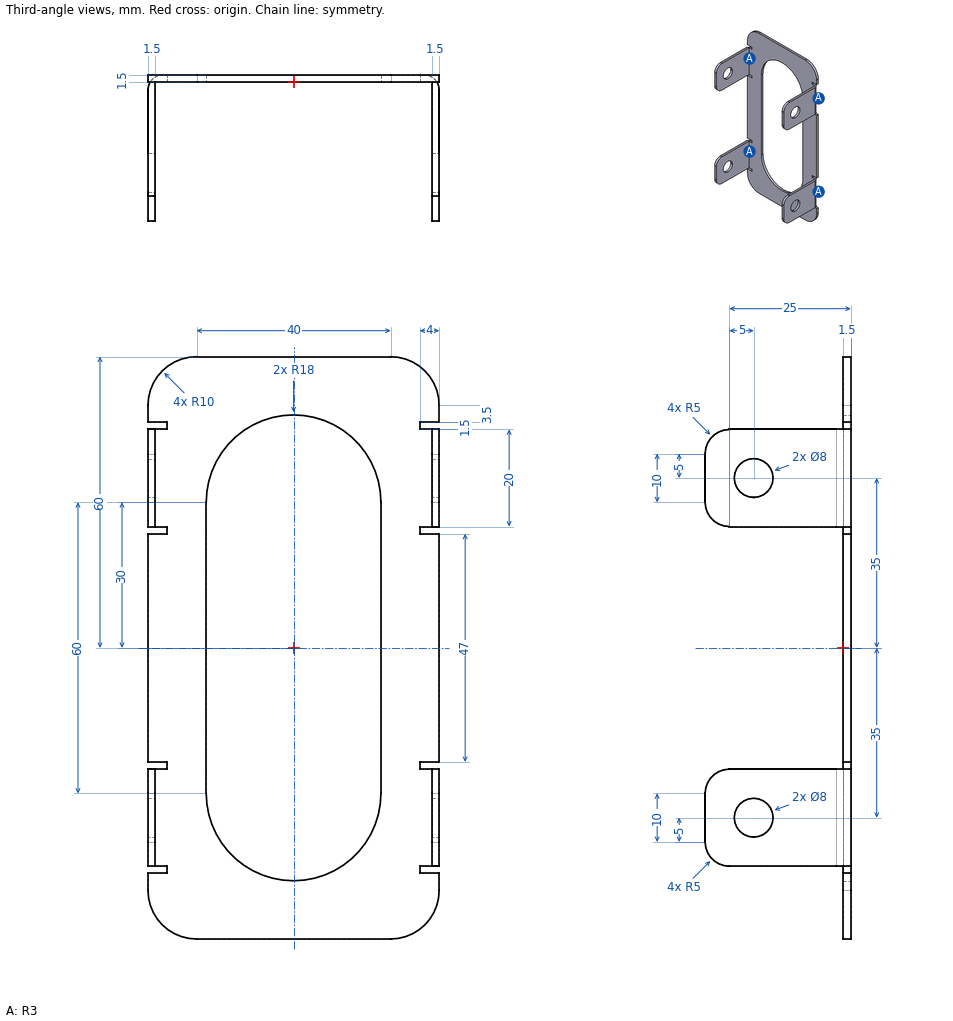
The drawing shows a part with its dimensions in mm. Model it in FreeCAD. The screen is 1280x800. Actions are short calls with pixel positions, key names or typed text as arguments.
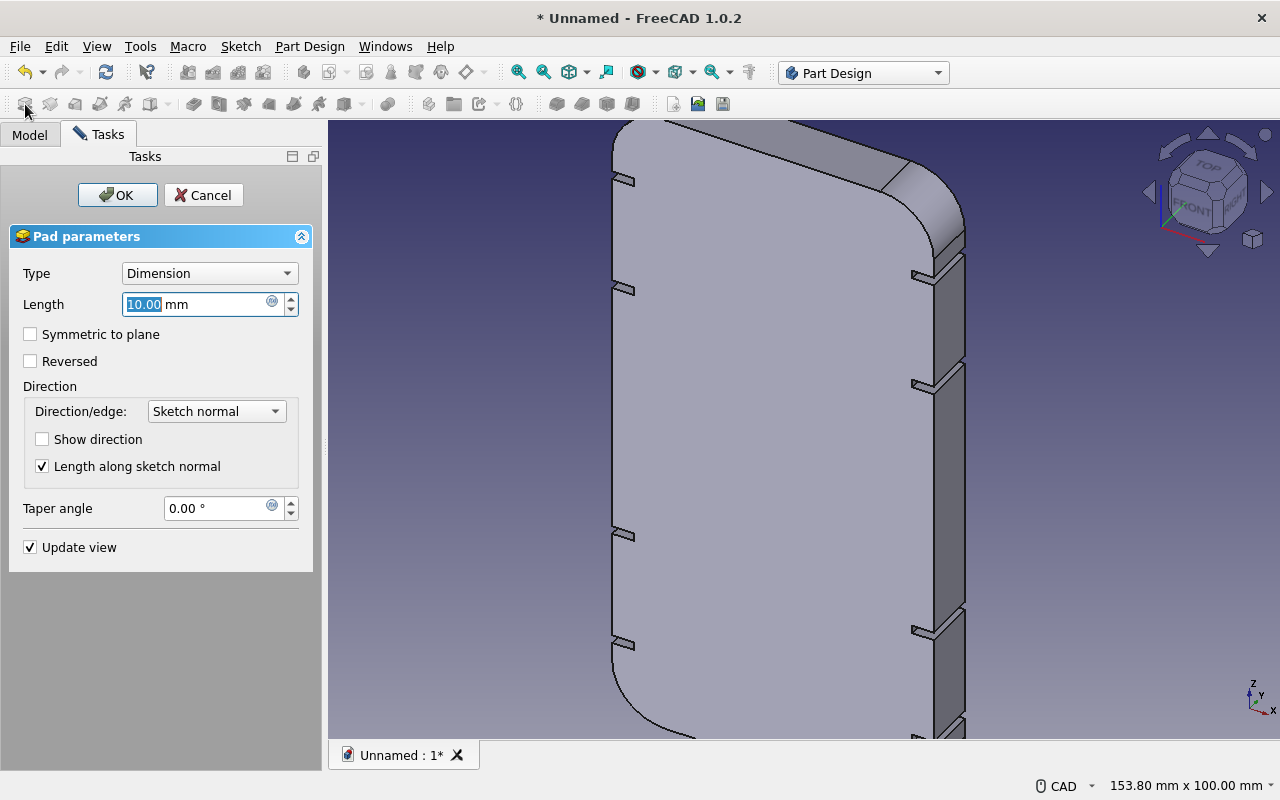
text(1.5)
key(Tab)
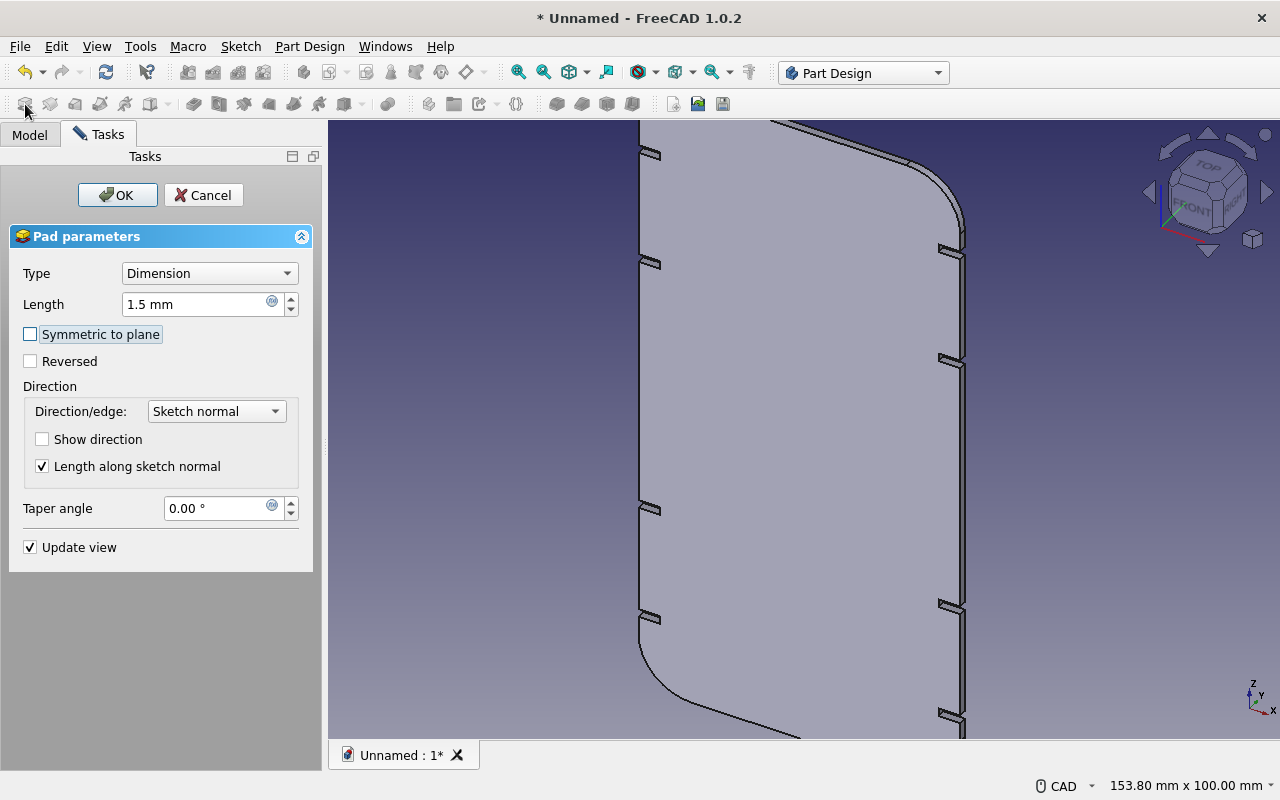
click(31, 361)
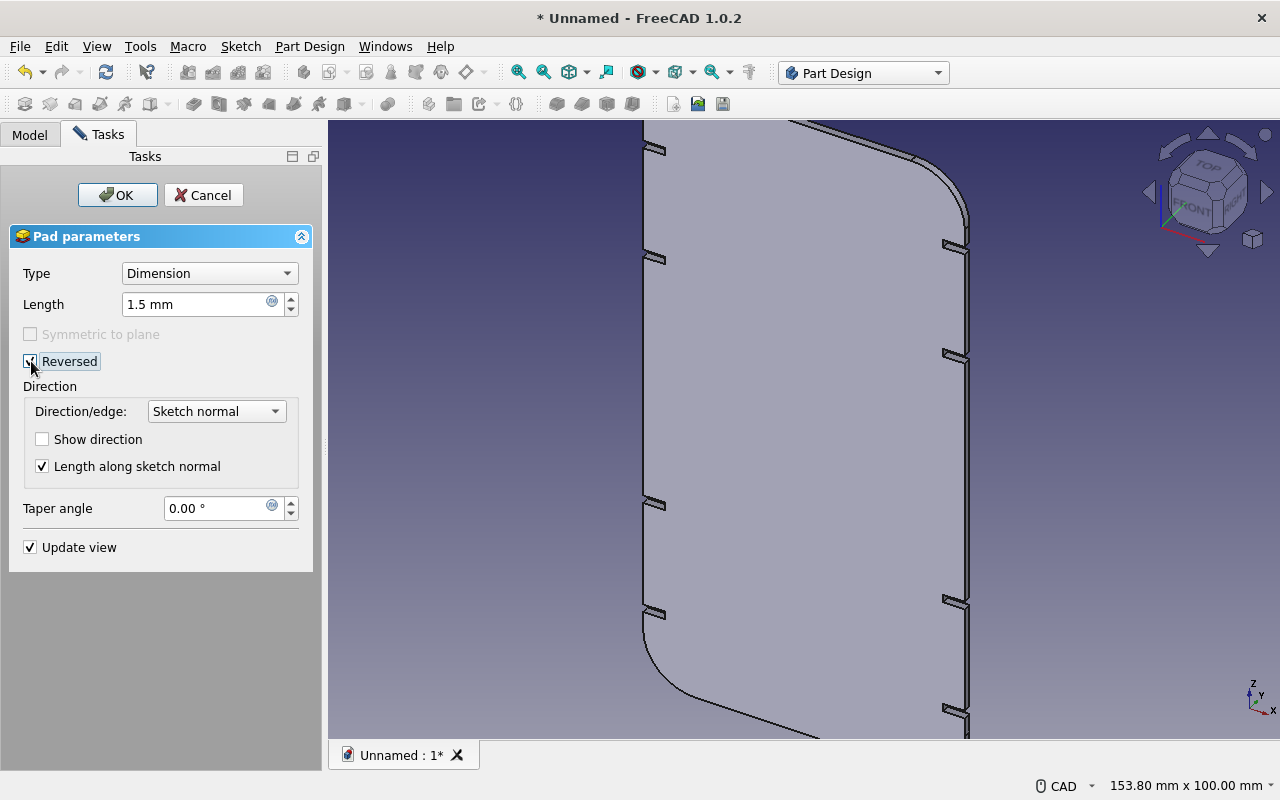
click(118, 195)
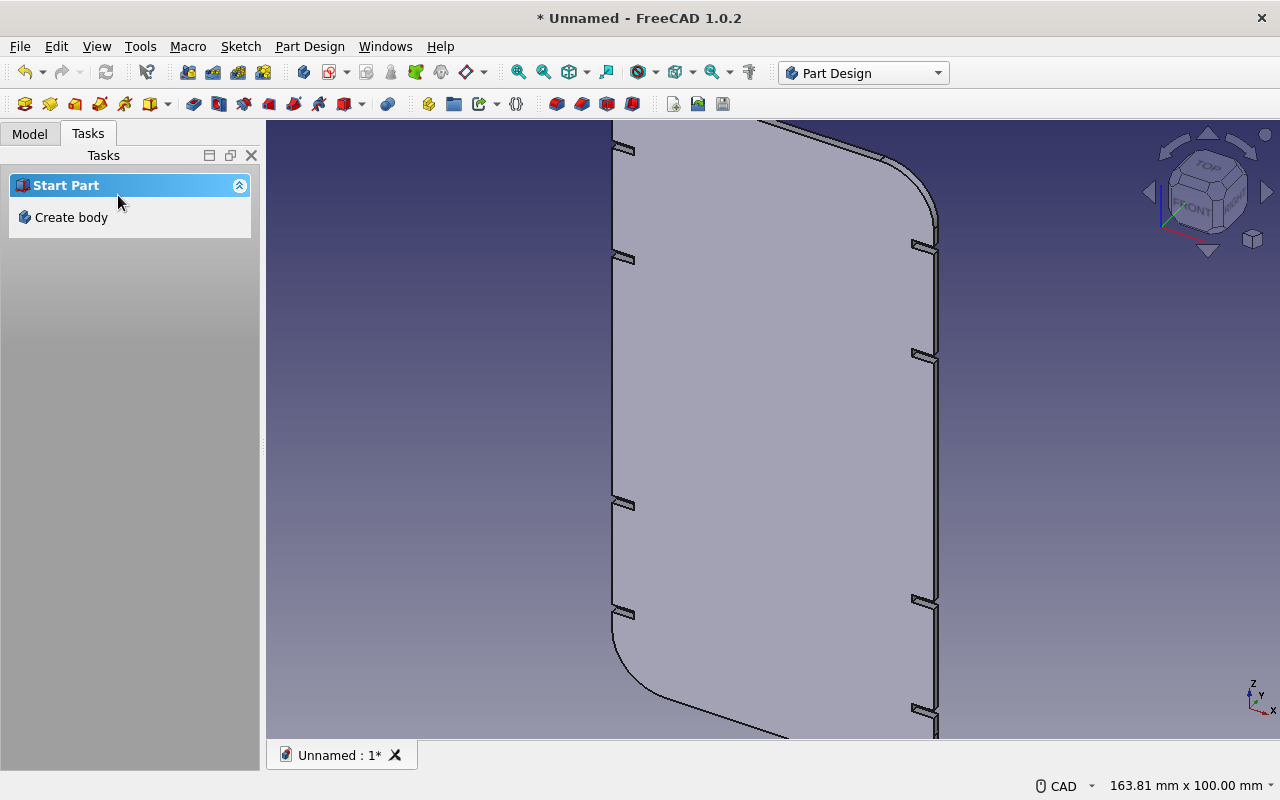
click(519, 72)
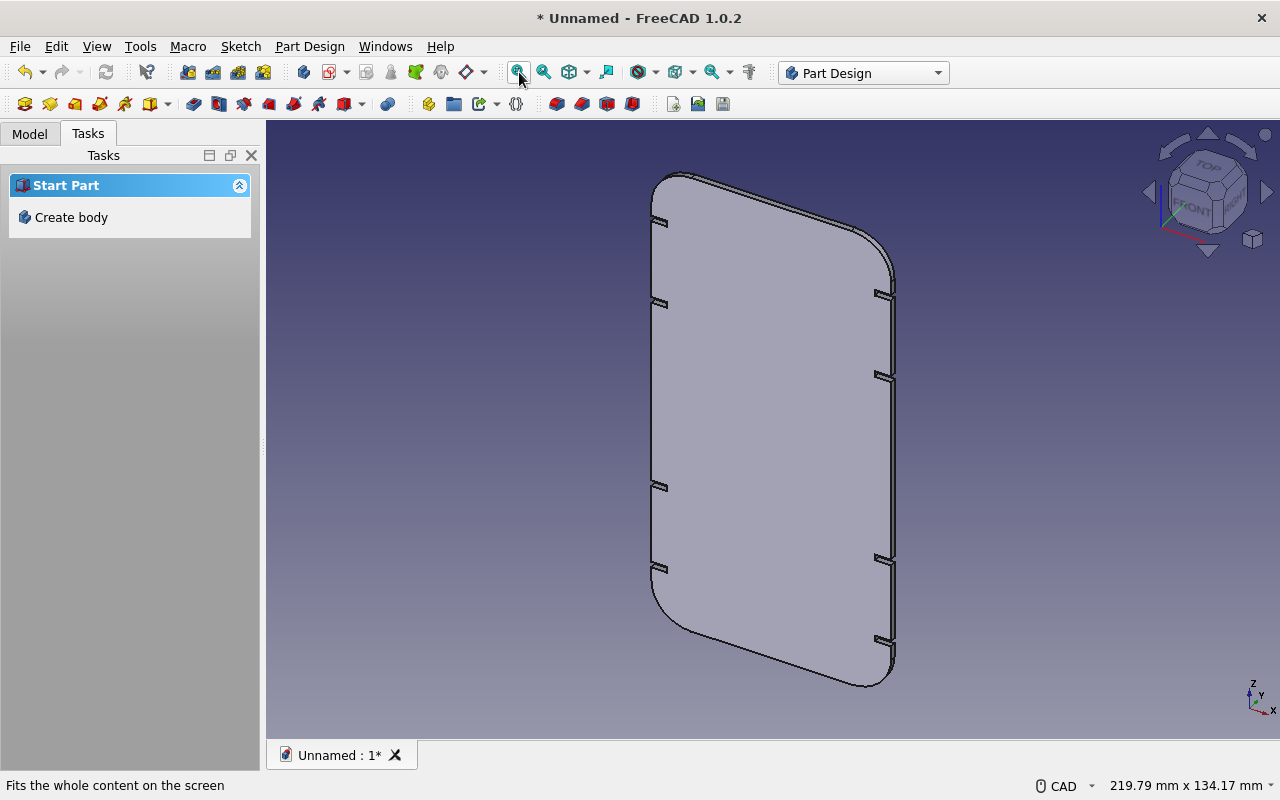
scroll(893, 392, up, 7)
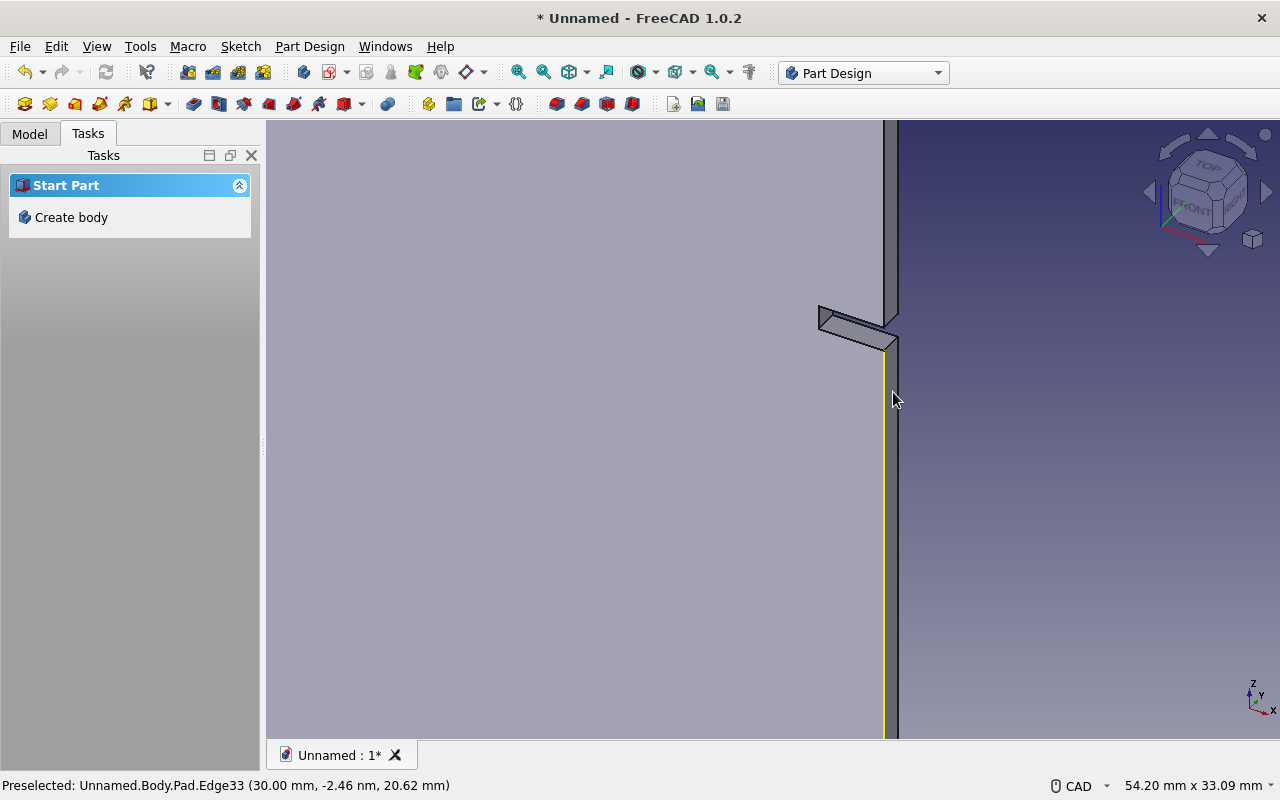
click(519, 72)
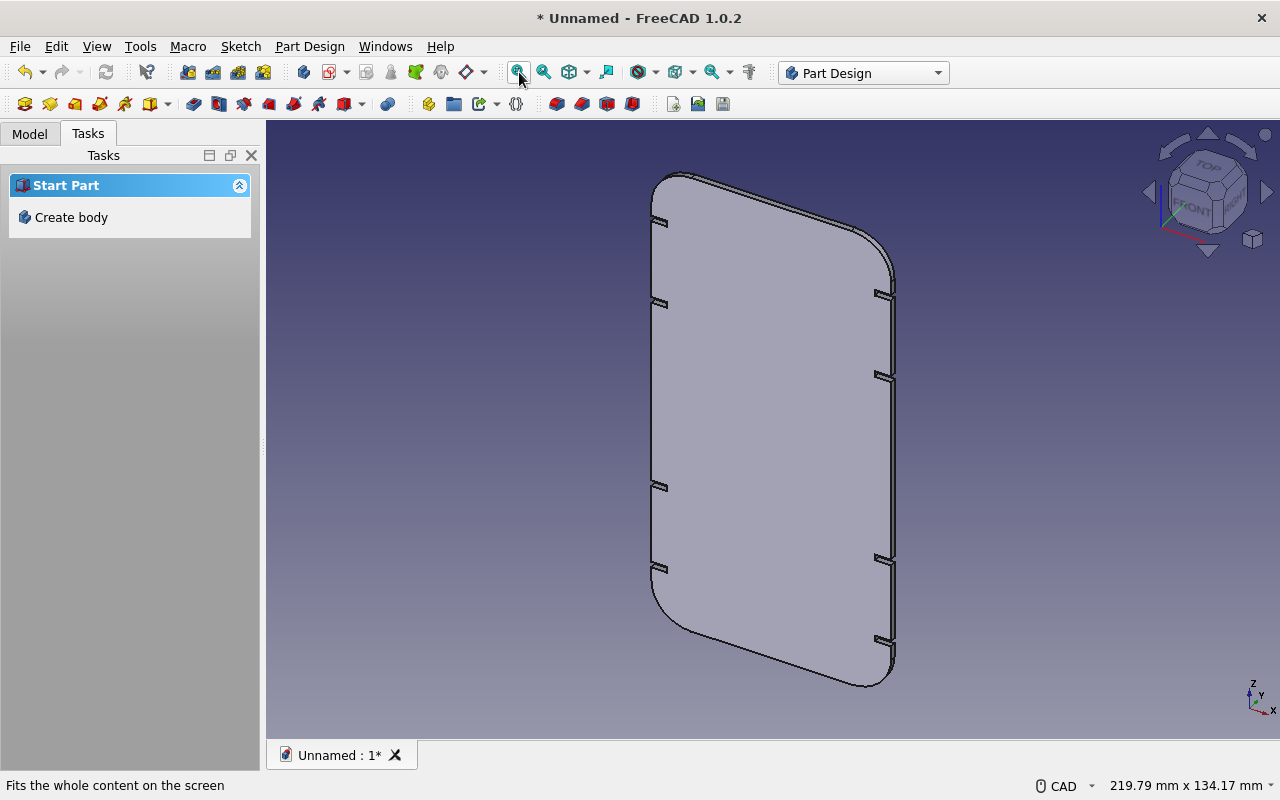
key(0)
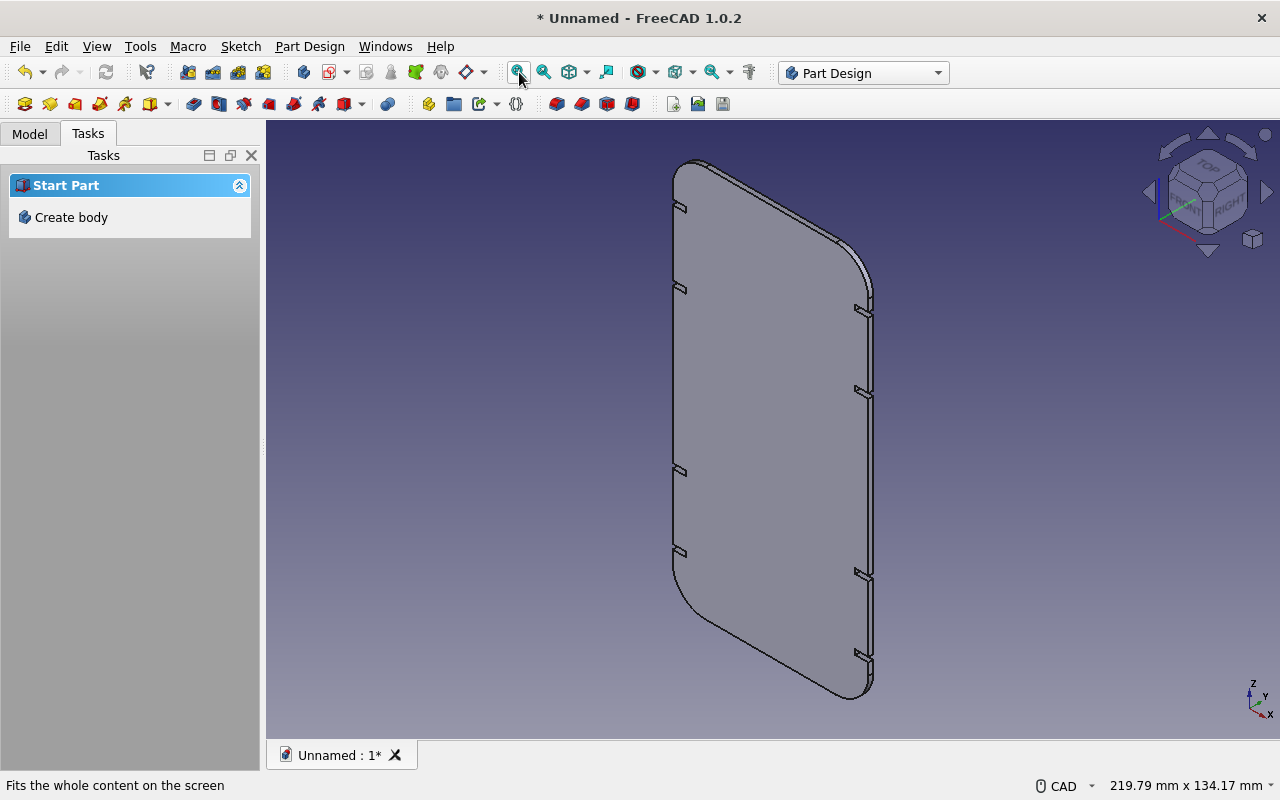
scroll(871, 409, up, 7)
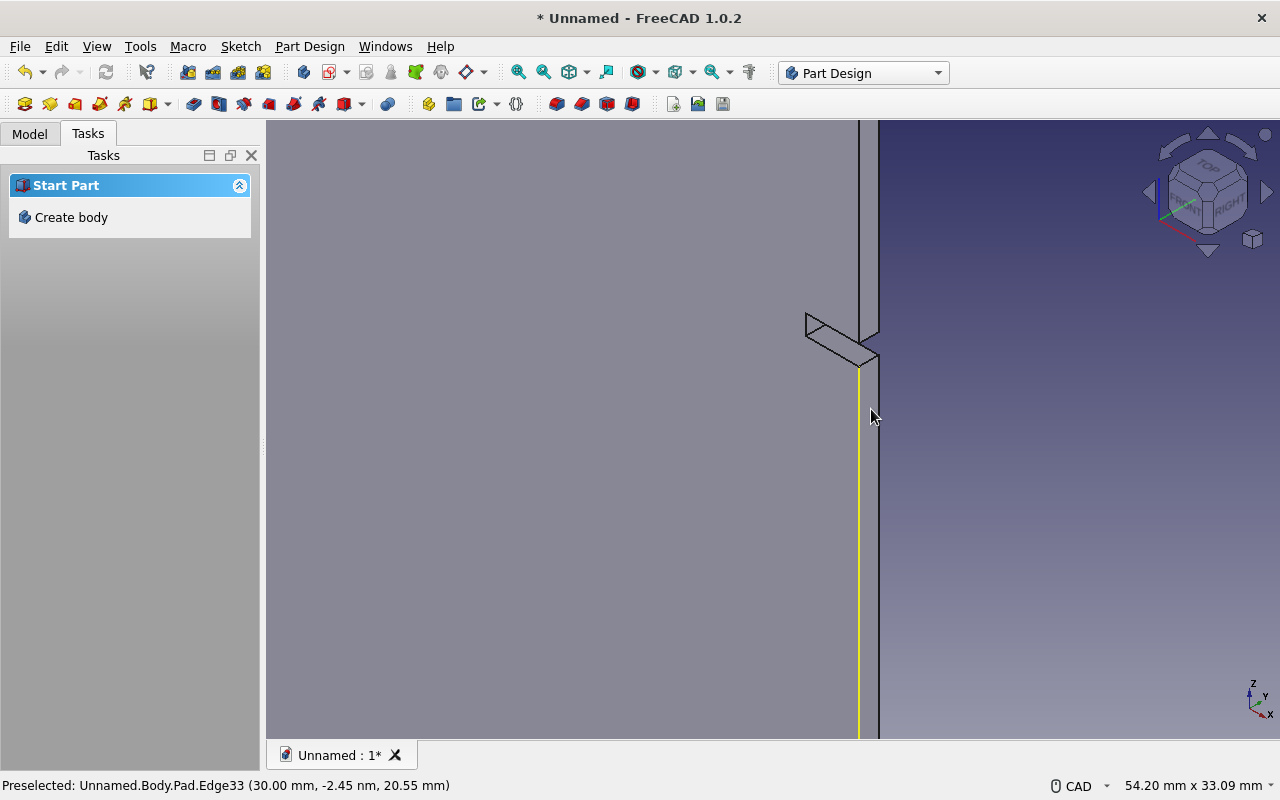
click(869, 411)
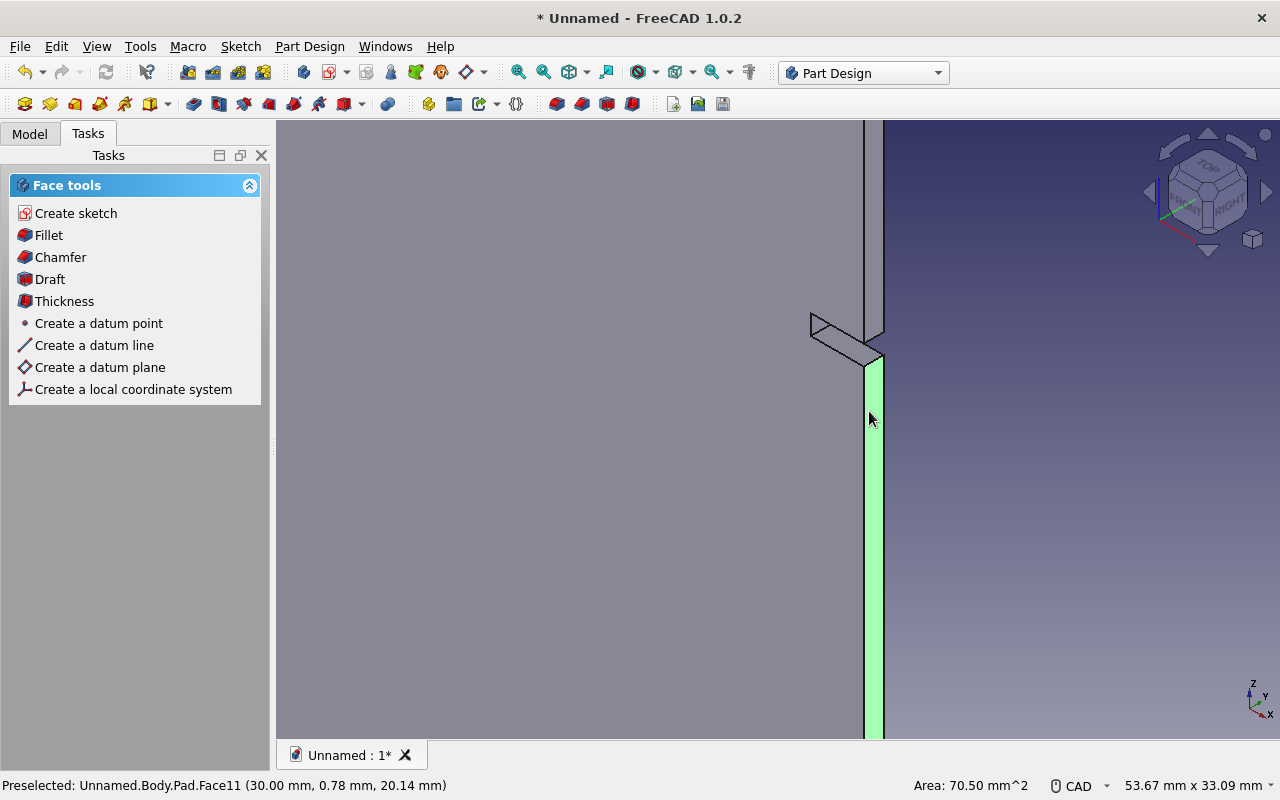
click(328, 72)